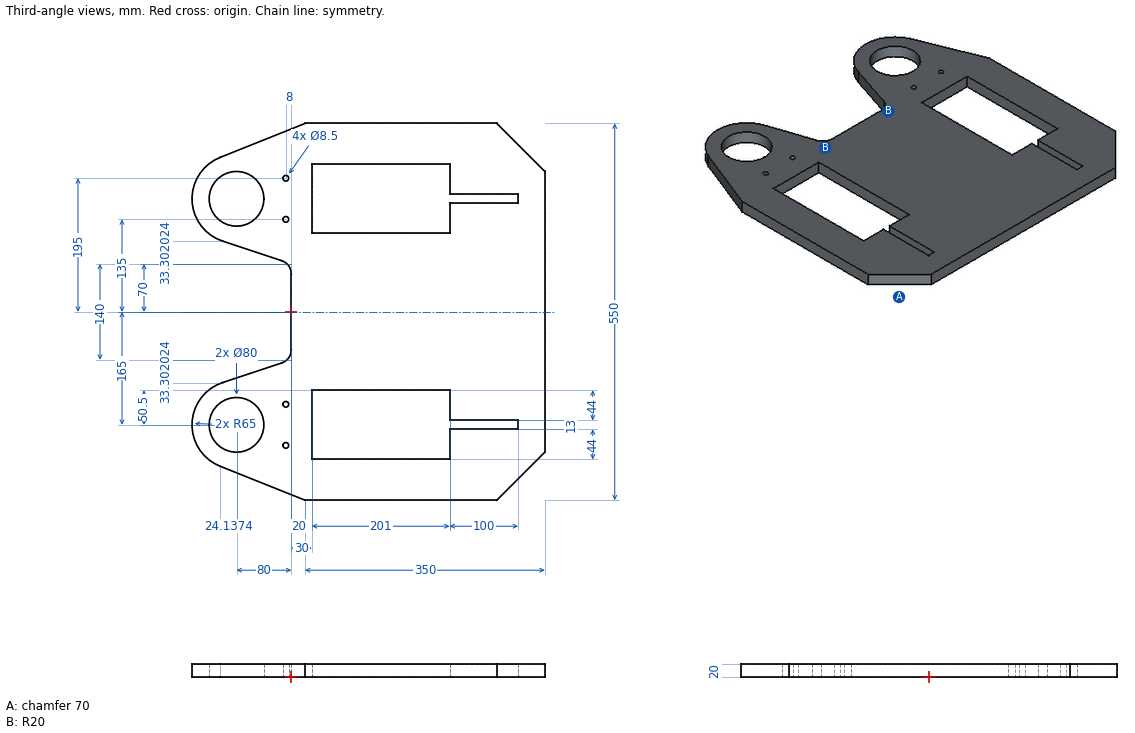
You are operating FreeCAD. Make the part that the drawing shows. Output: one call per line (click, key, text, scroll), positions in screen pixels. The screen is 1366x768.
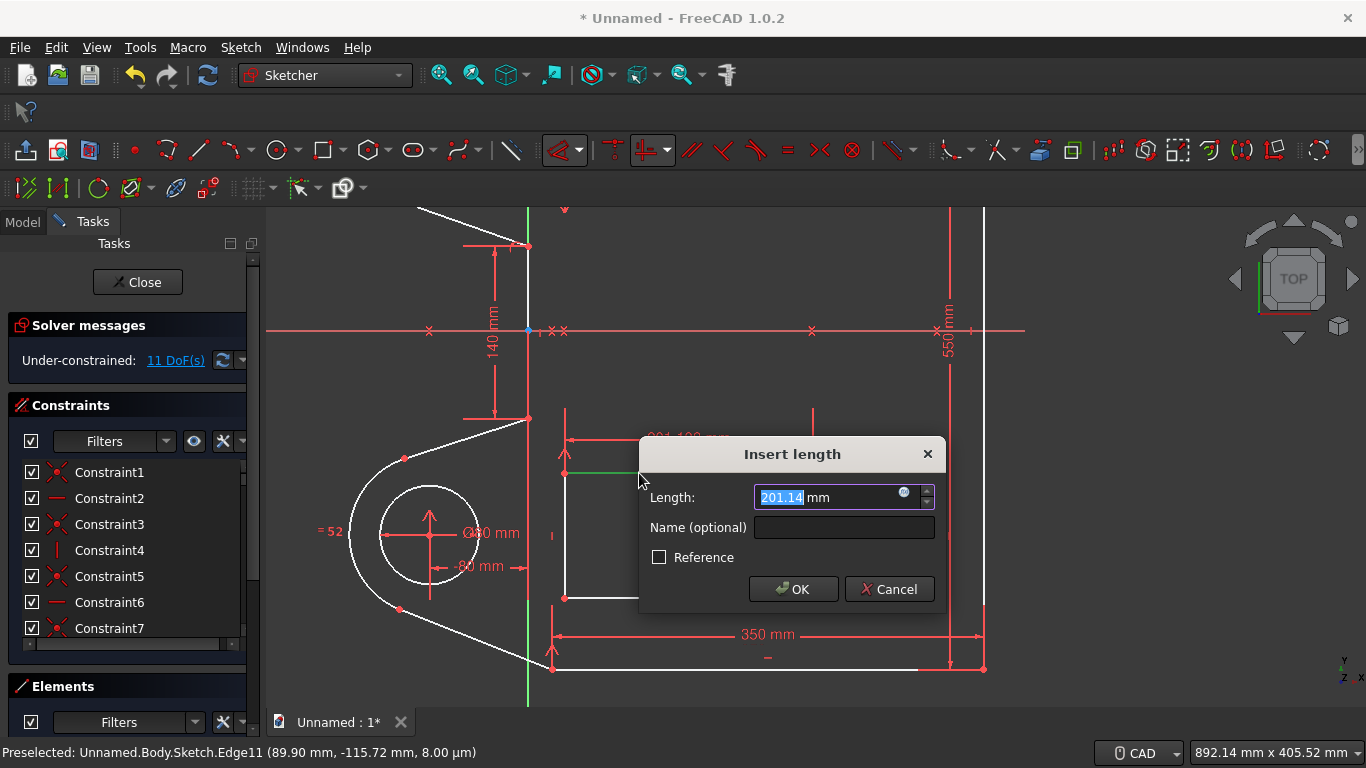
text(201)
key(Return)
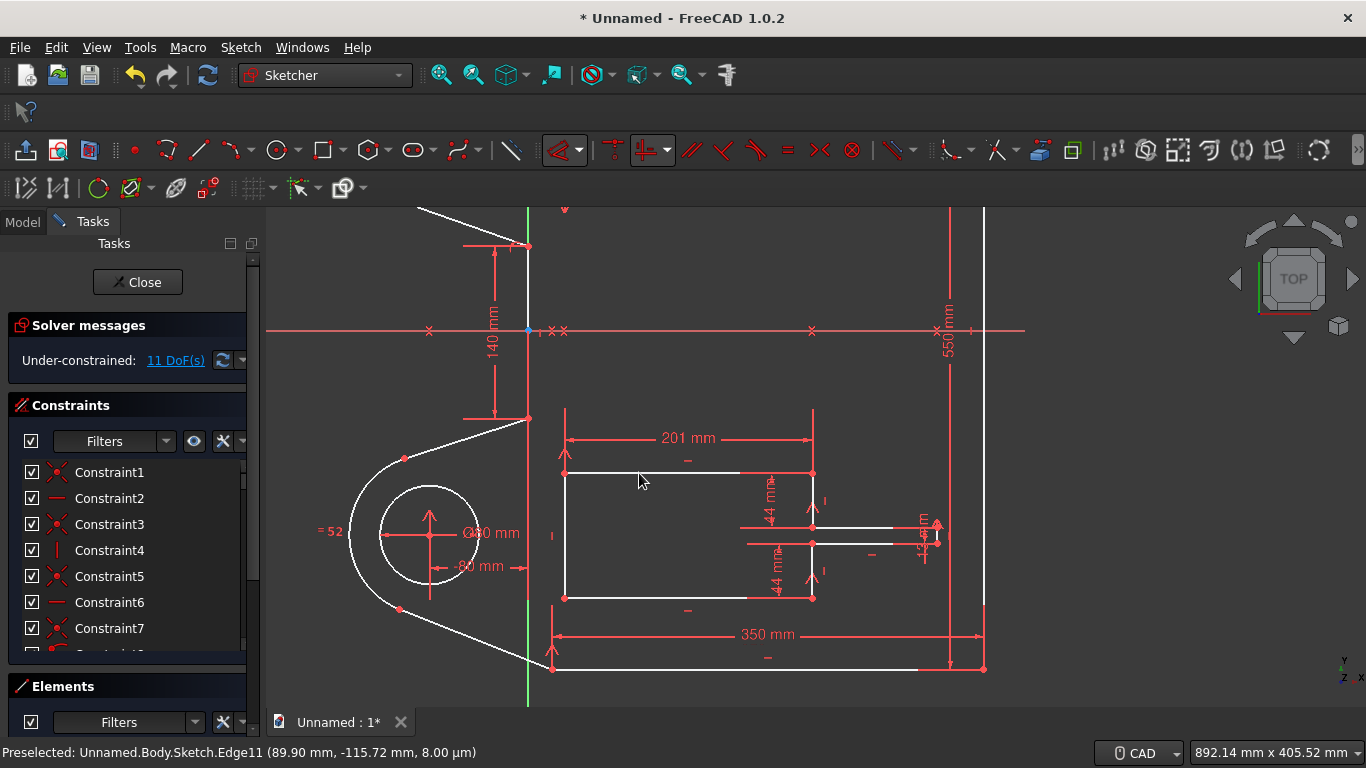
click(850, 528)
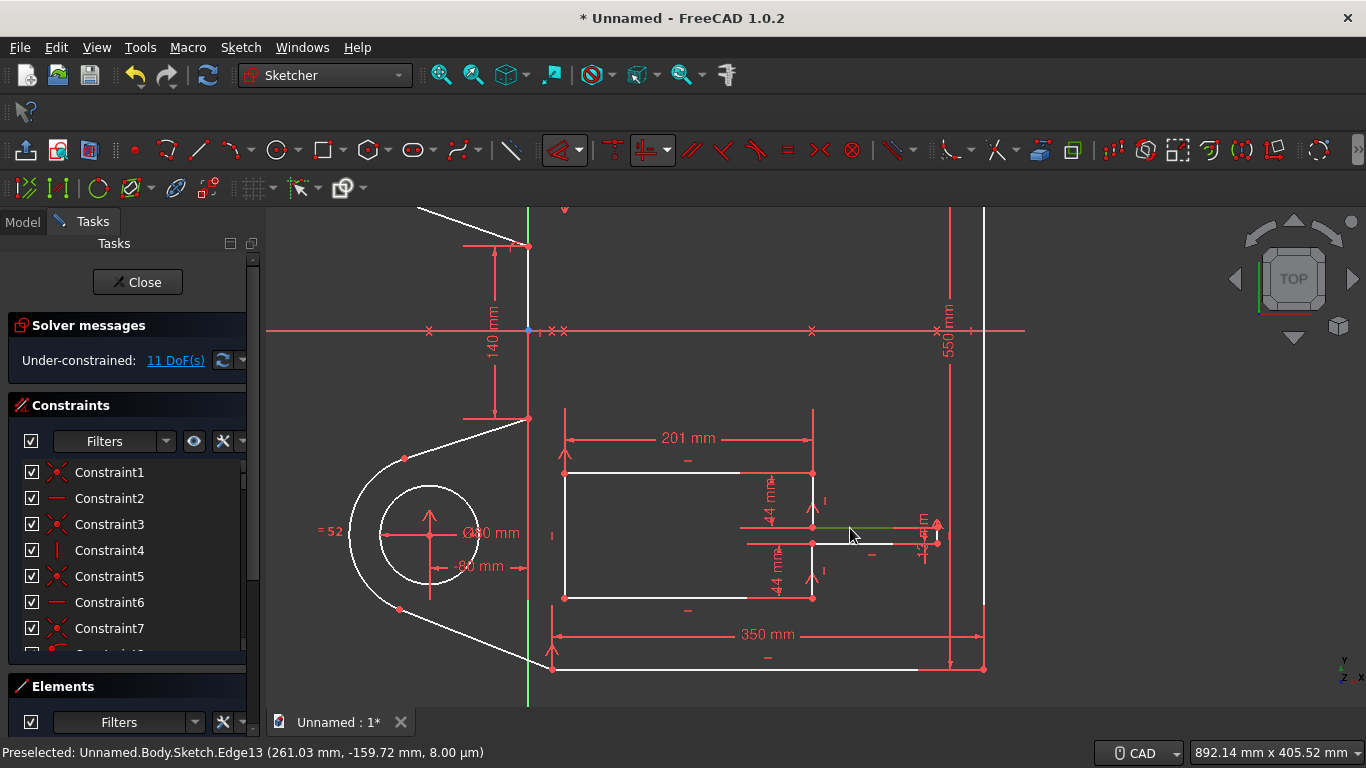
key(l)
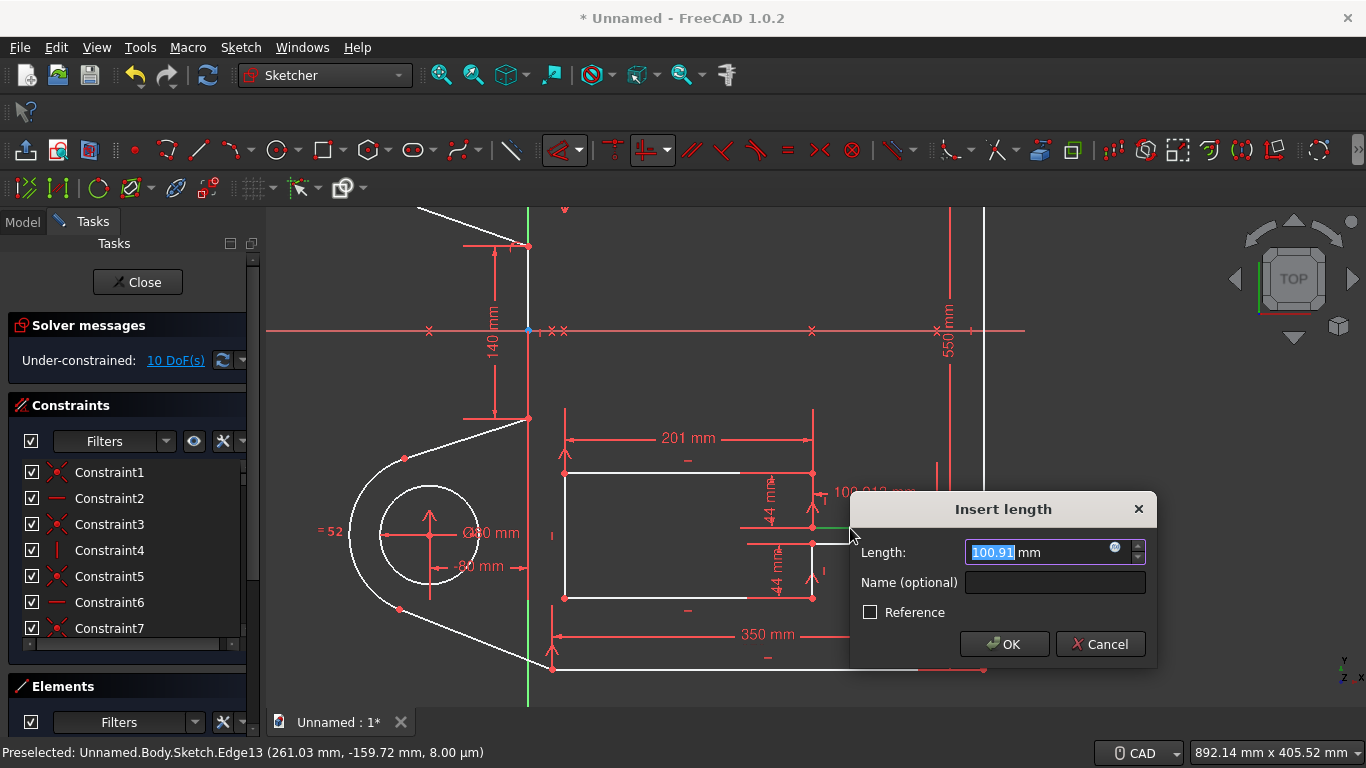
text(100)
key(Return)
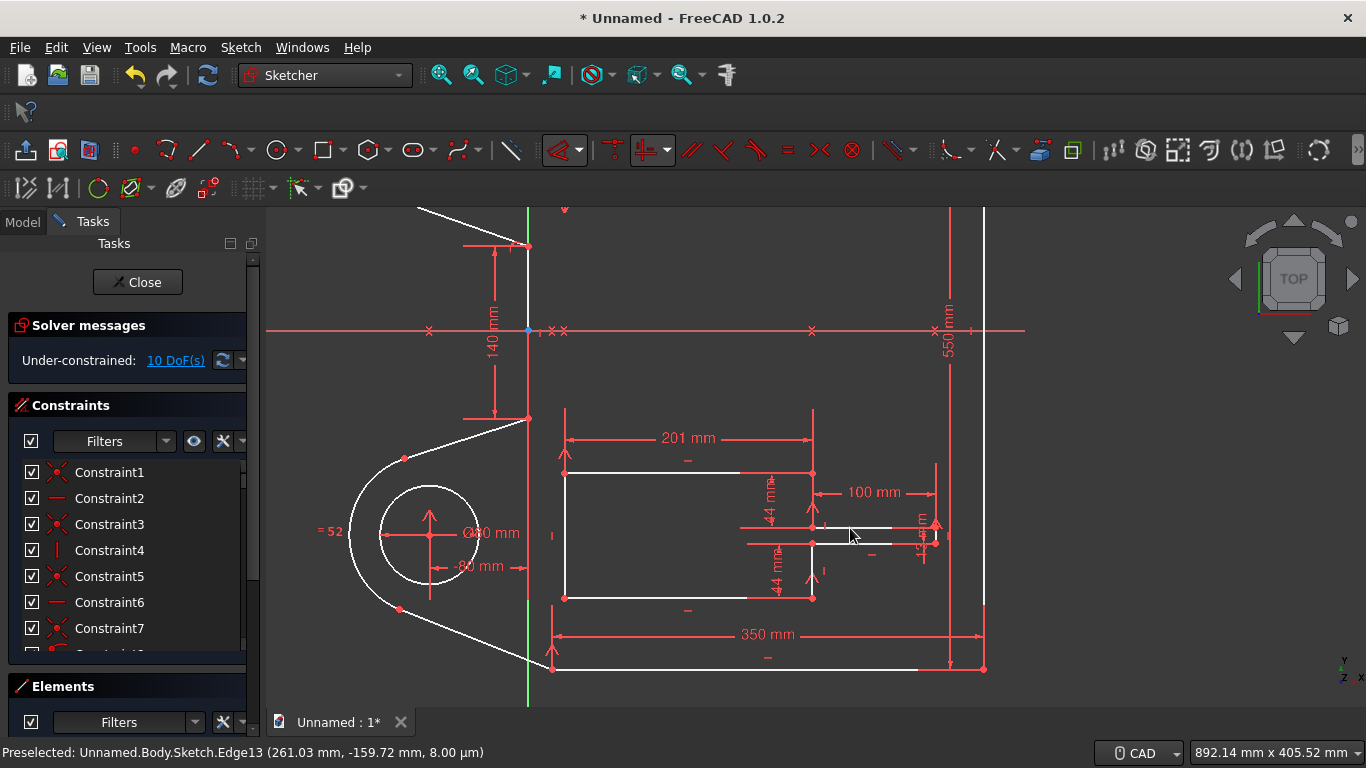
click(899, 544)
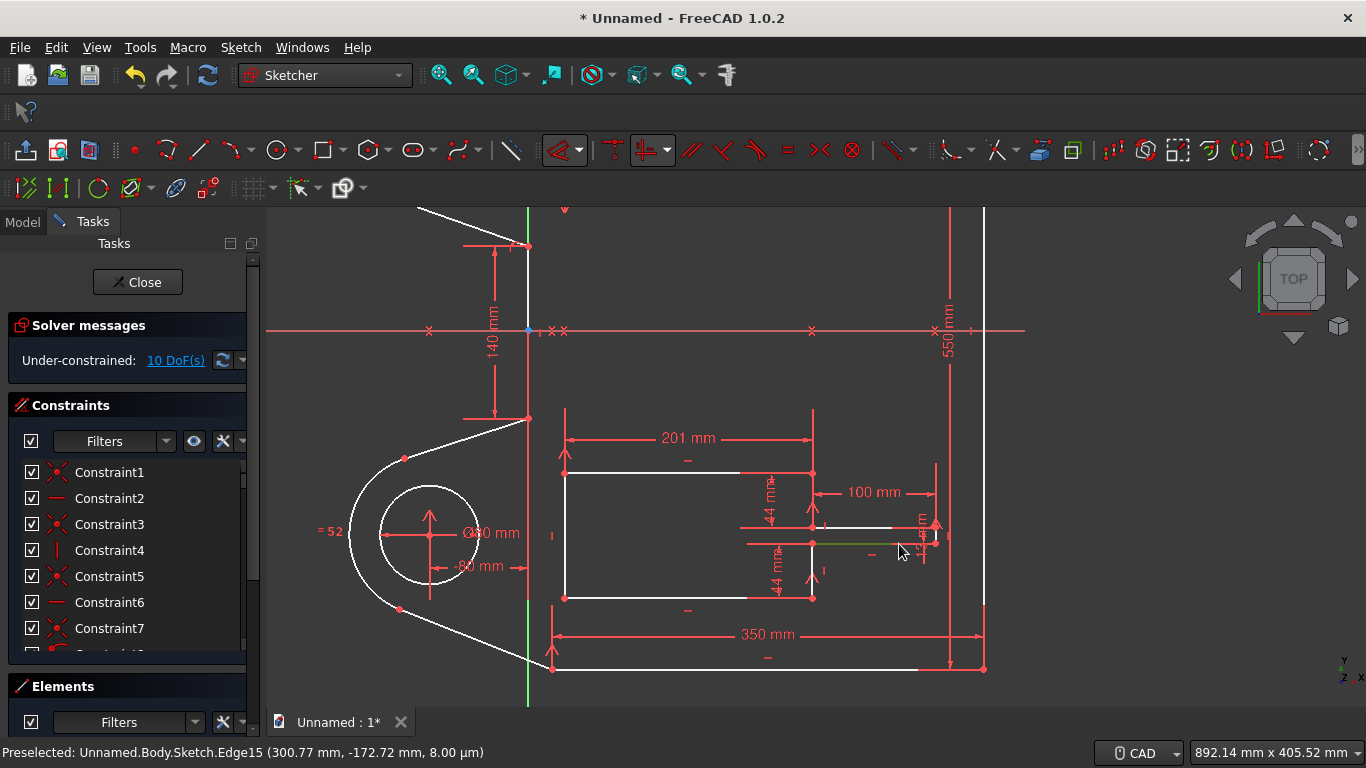
key(l)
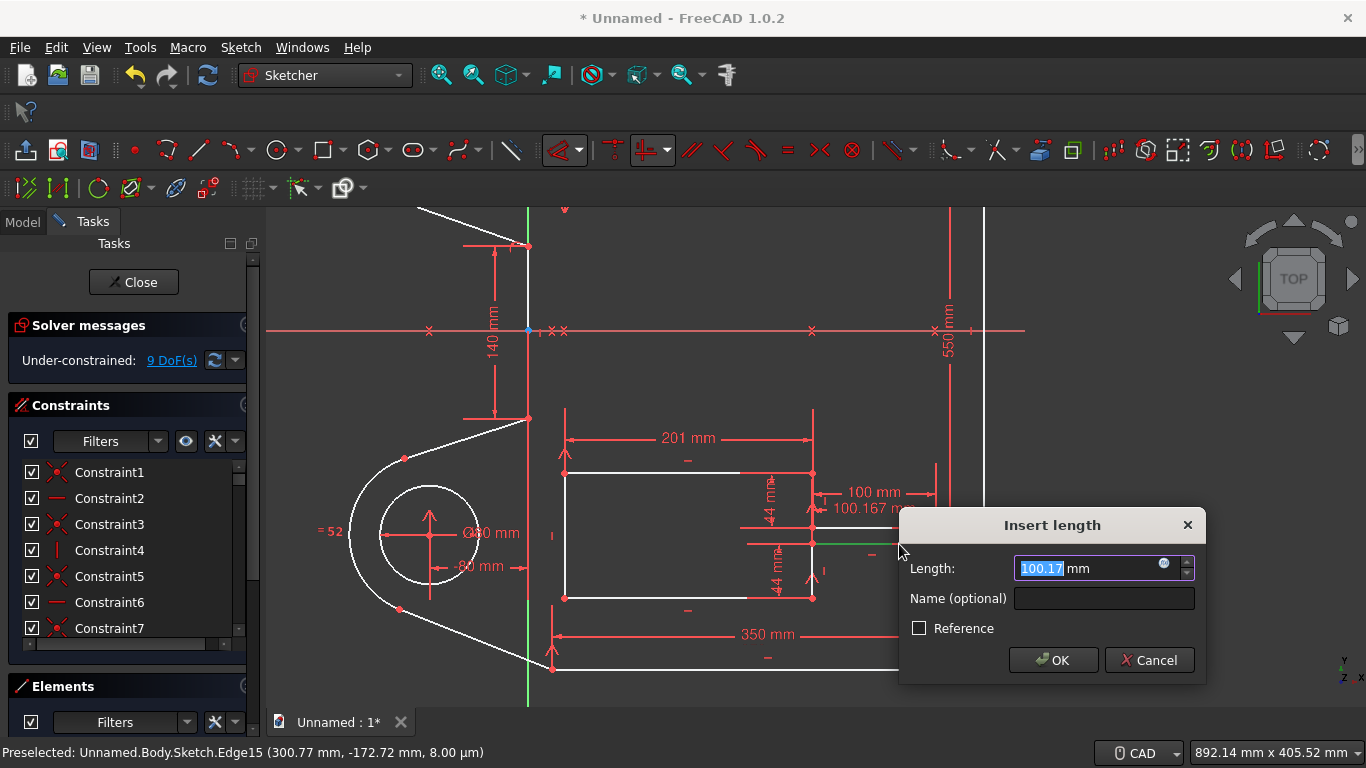
text(100)
key(Return)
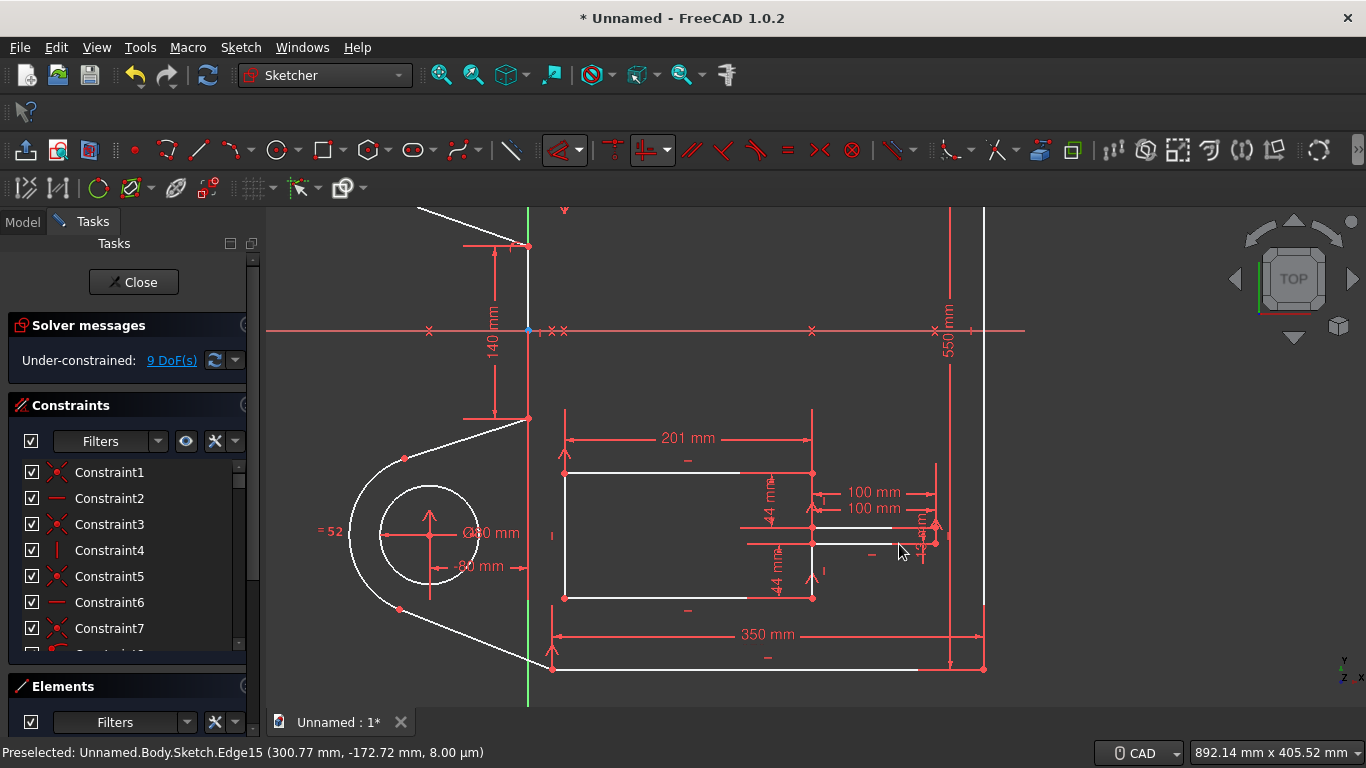
scroll(552, 670, up, 3)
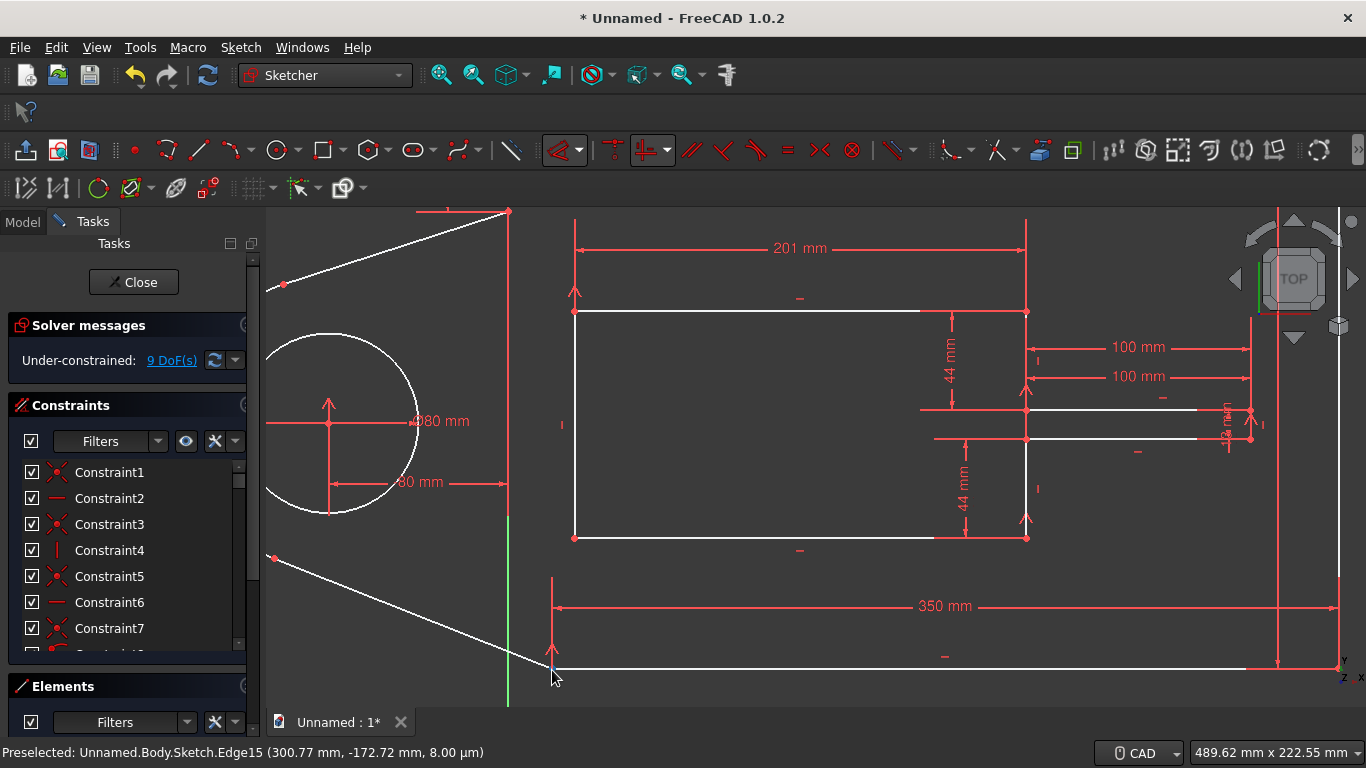
click(552, 669)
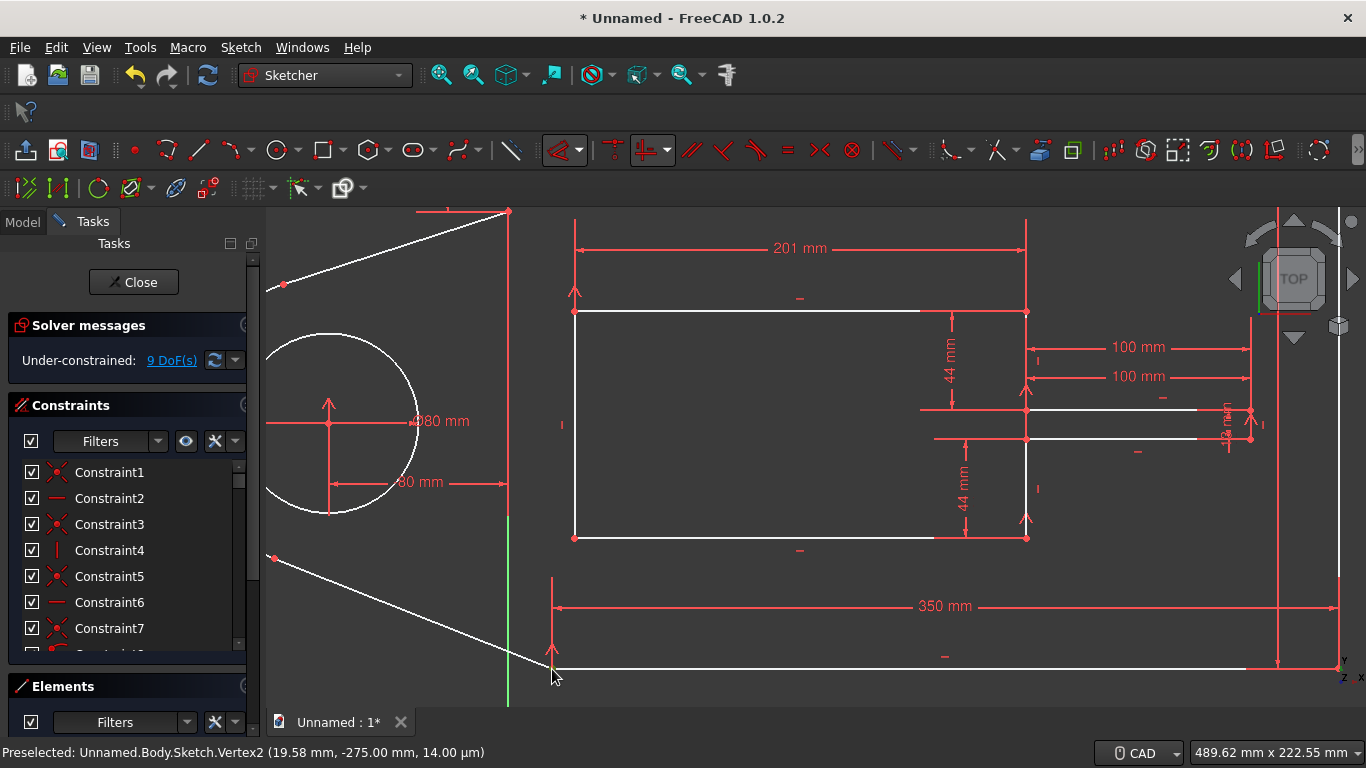
click(582, 150)